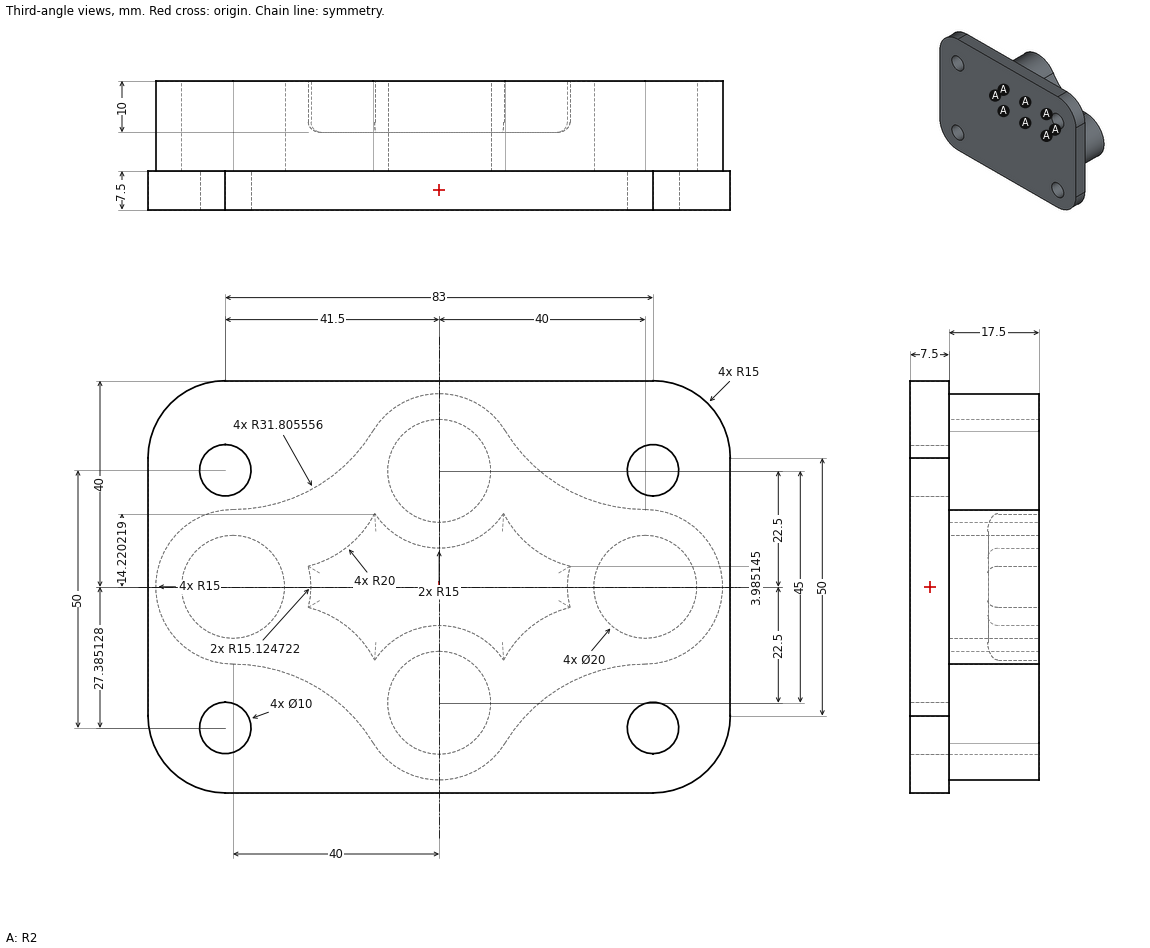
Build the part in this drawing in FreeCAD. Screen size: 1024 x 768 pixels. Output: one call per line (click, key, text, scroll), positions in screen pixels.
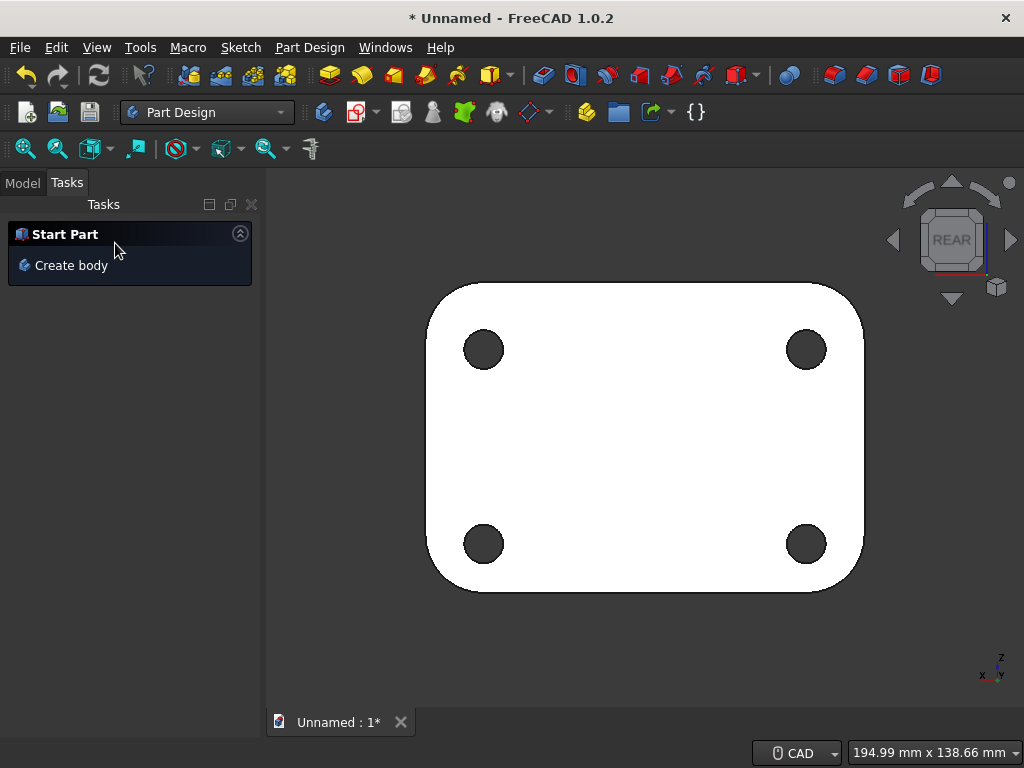
click(645, 436)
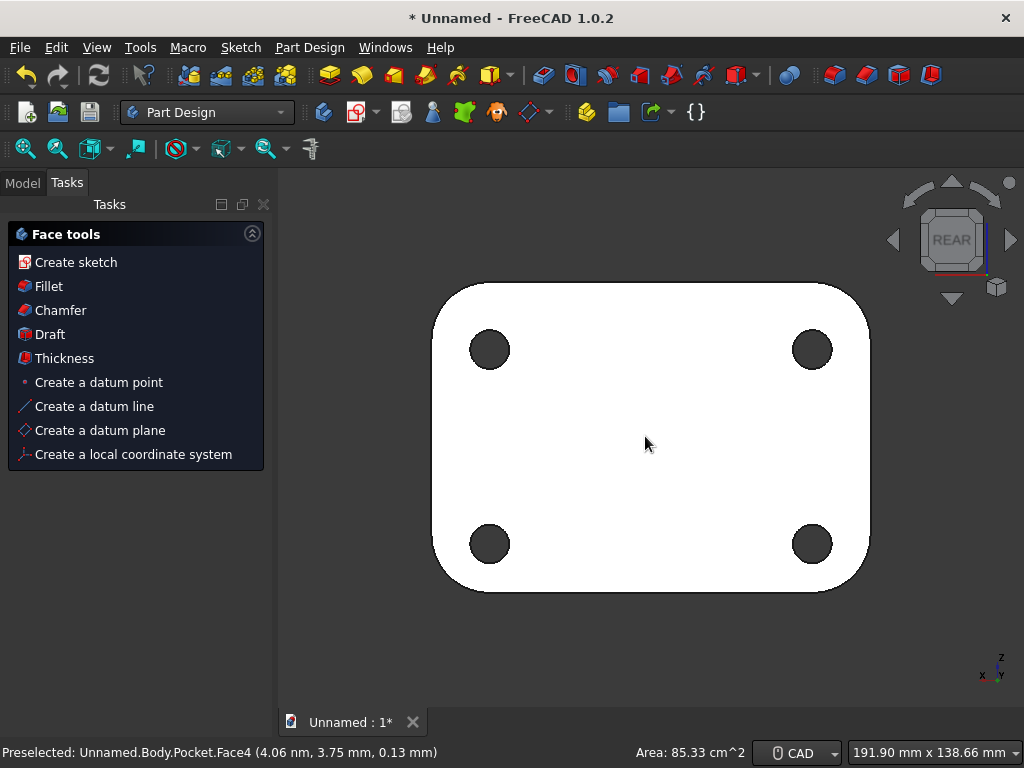
click(356, 112)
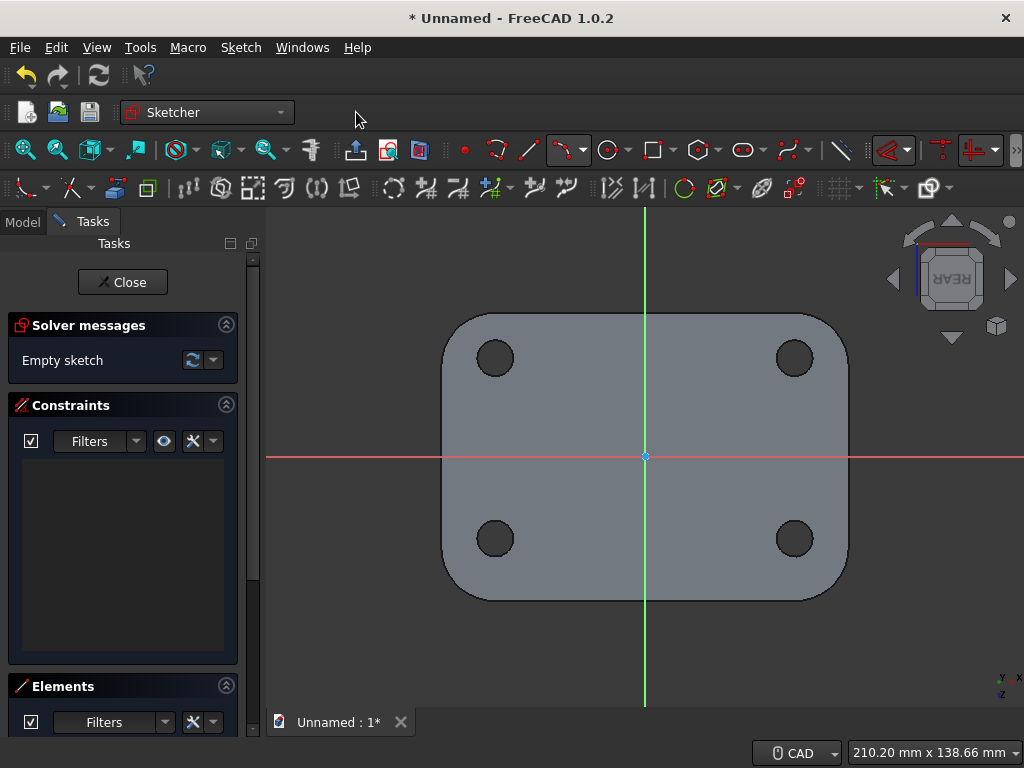
scroll(294, 457, down, 1)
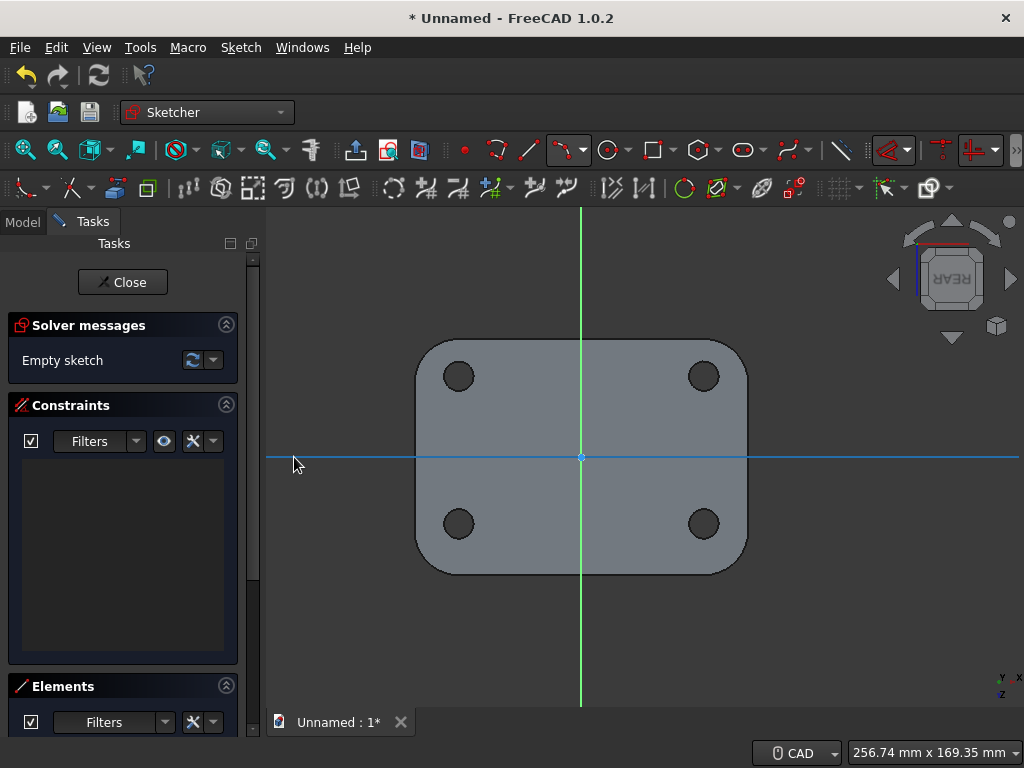
click(562, 150)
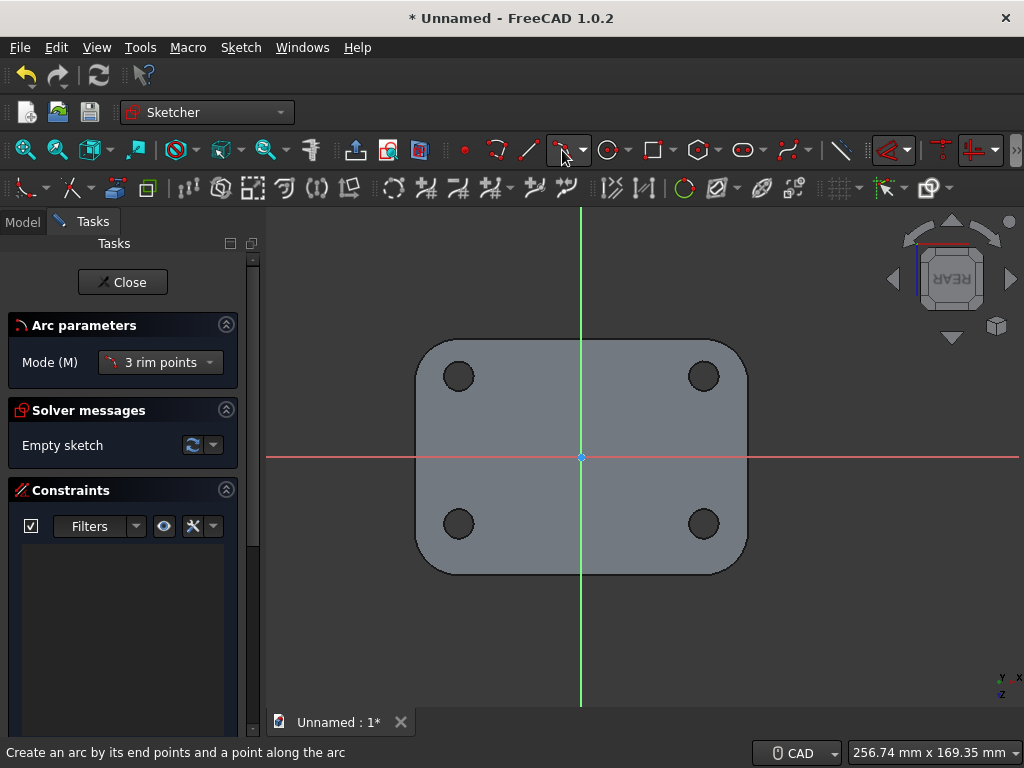
click(544, 547)
click(619, 547)
click(564, 564)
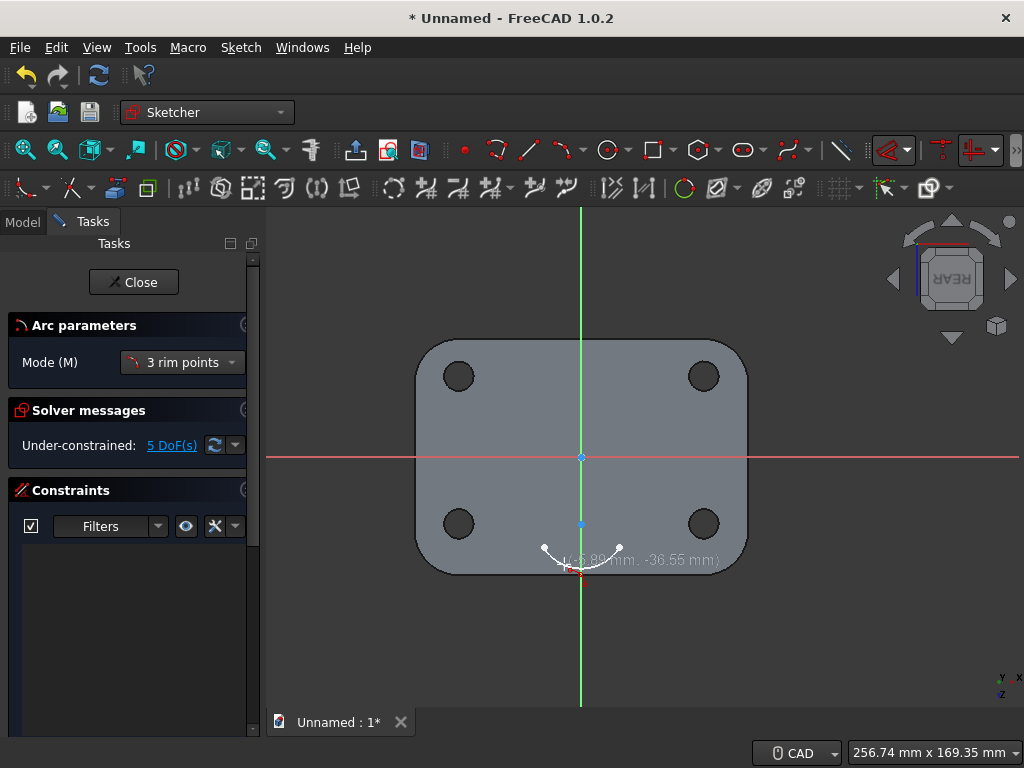
click(619, 548)
click(699, 501)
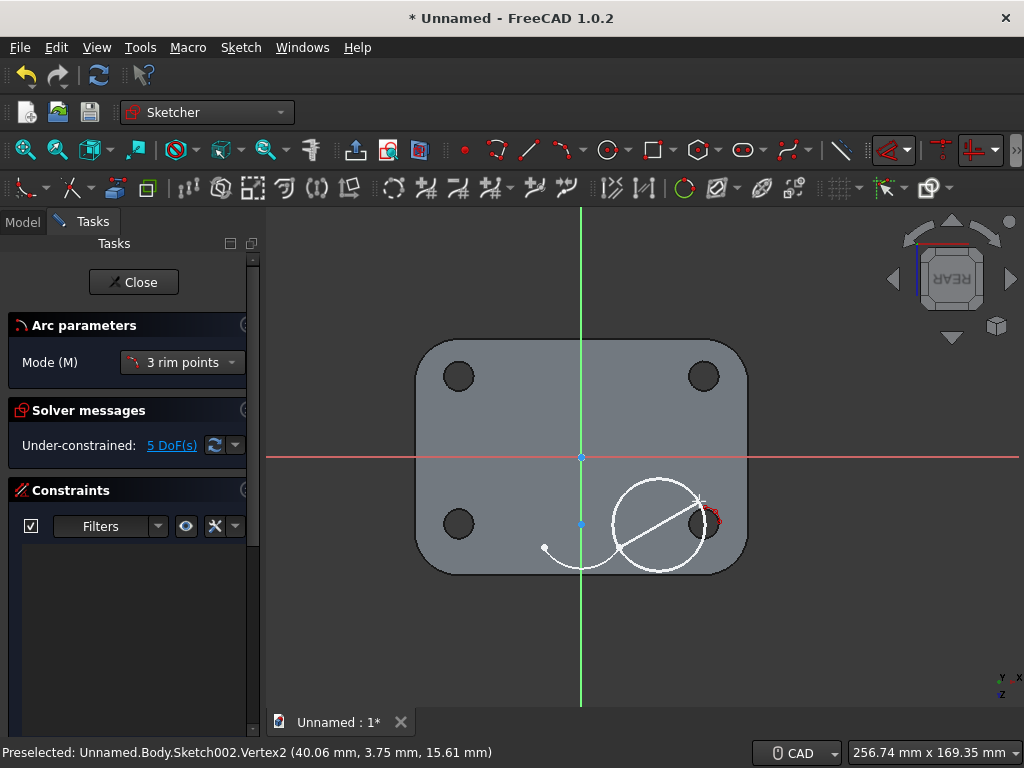
scroll(653, 513, up, 2)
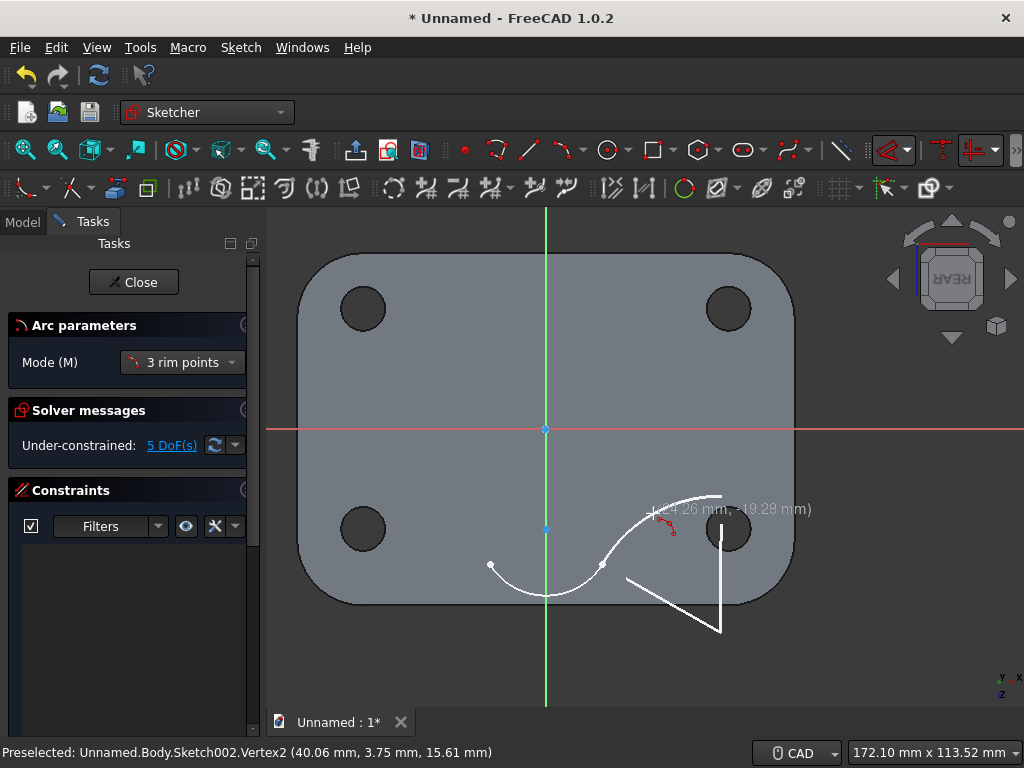
click(653, 513)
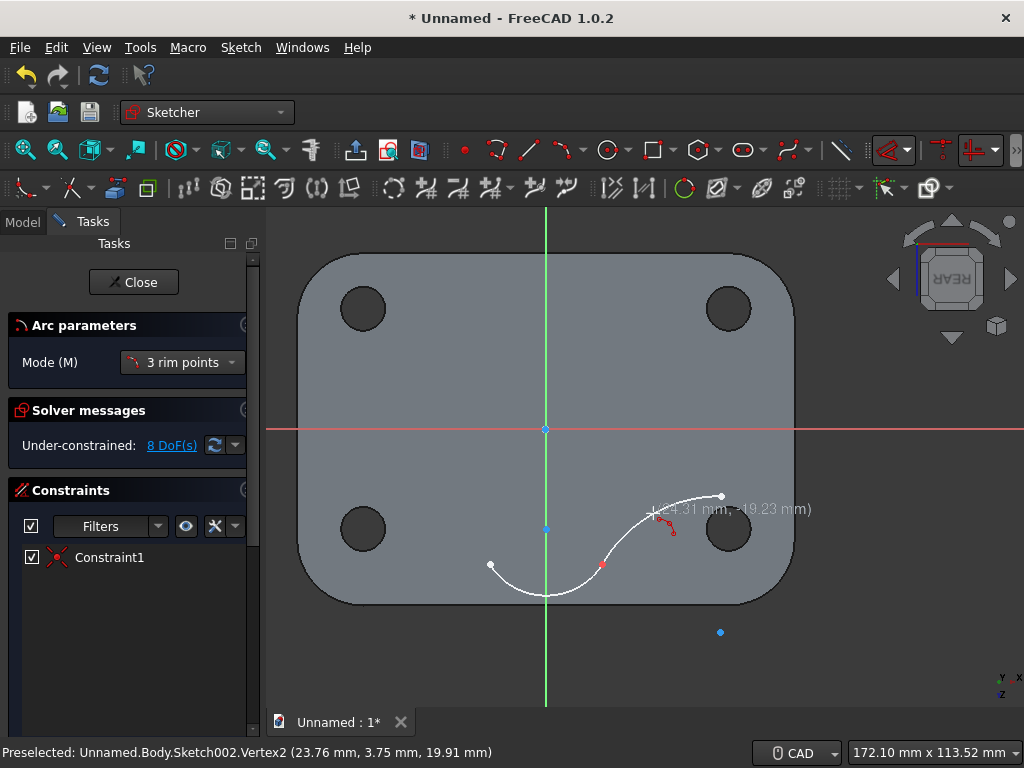
click(721, 496)
click(722, 363)
click(776, 468)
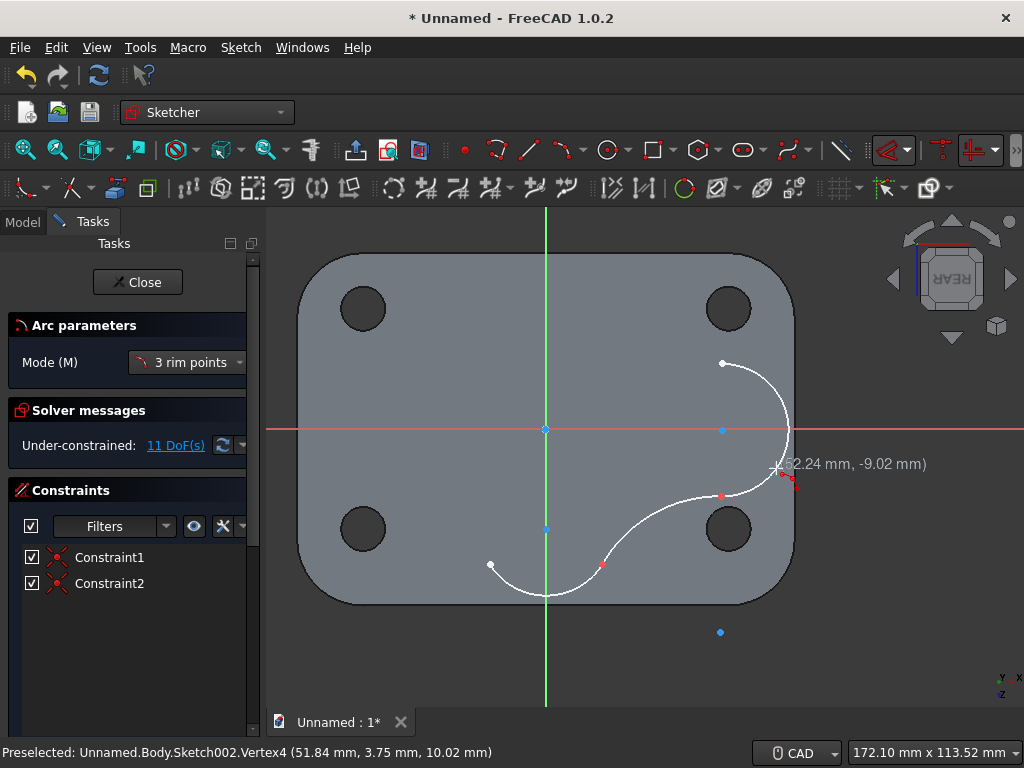
click(722, 364)
click(602, 296)
click(653, 345)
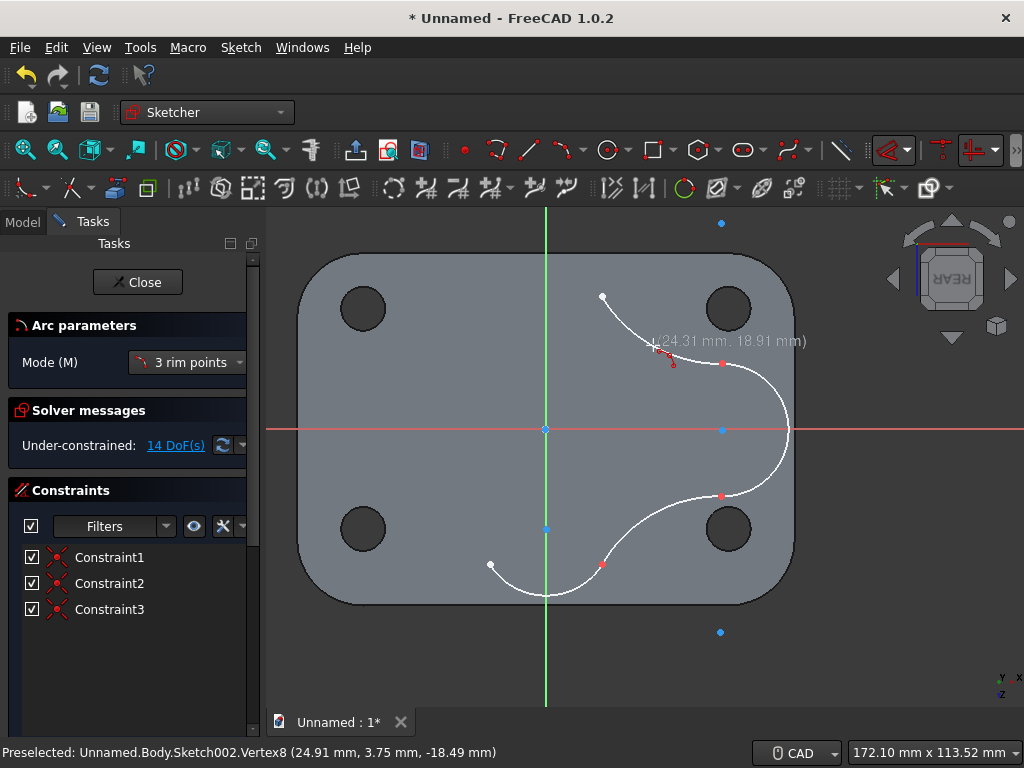
click(602, 297)
click(489, 296)
click(572, 270)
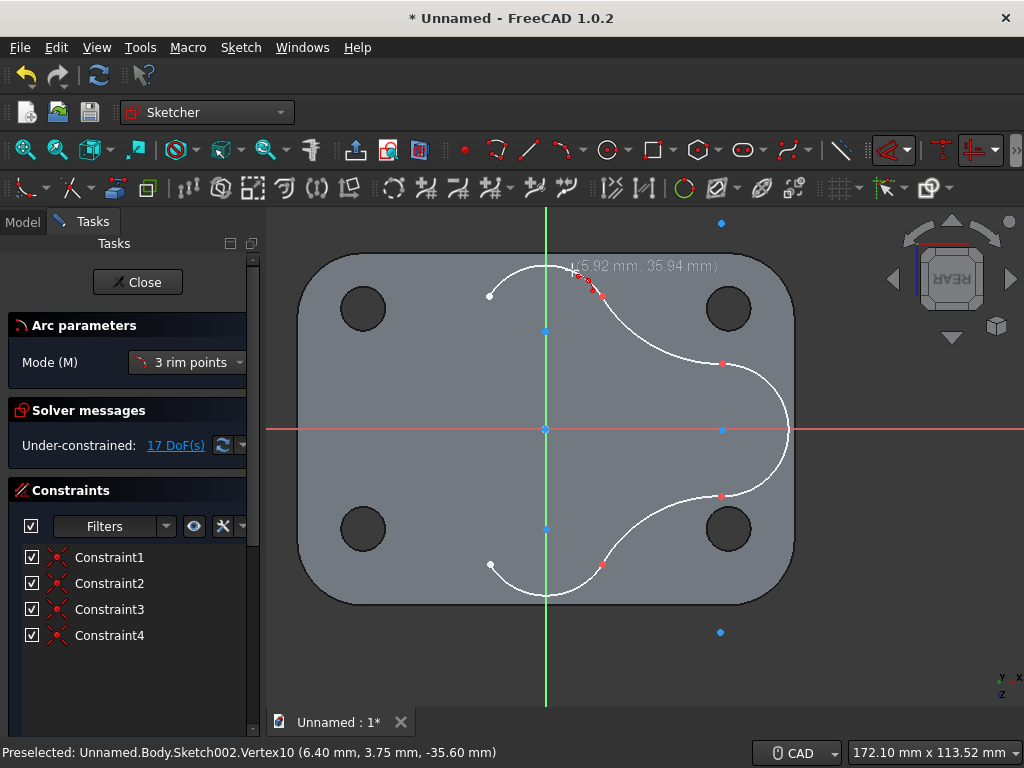
click(489, 297)
click(370, 363)
click(438, 345)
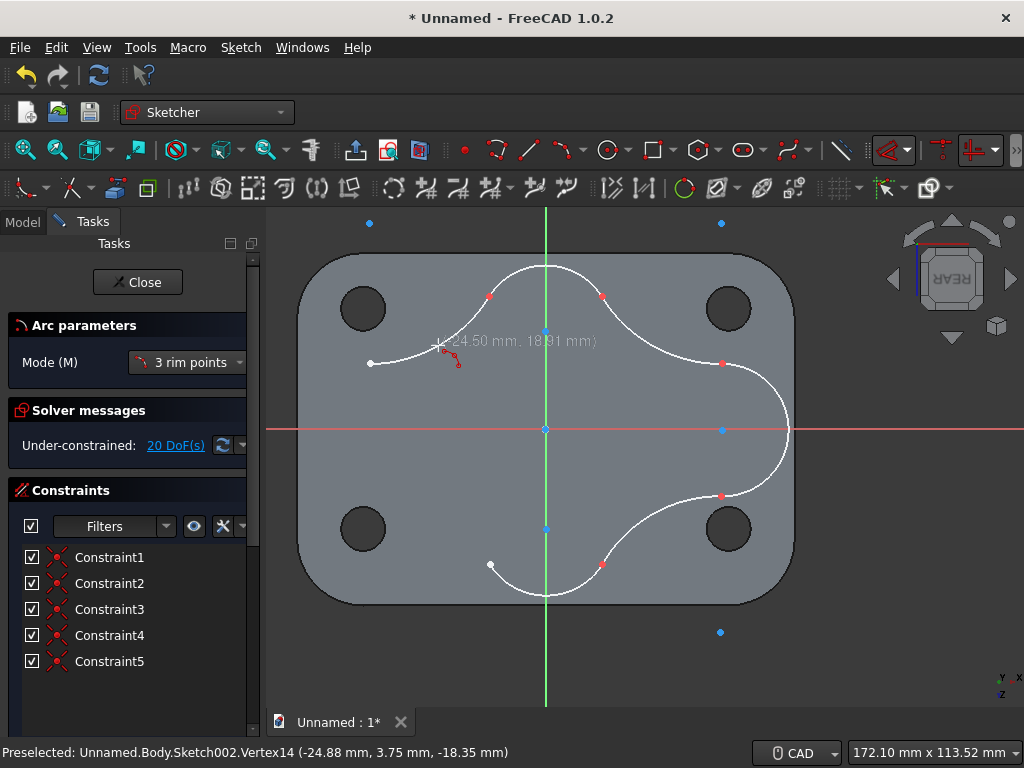
click(370, 364)
click(370, 495)
click(316, 390)